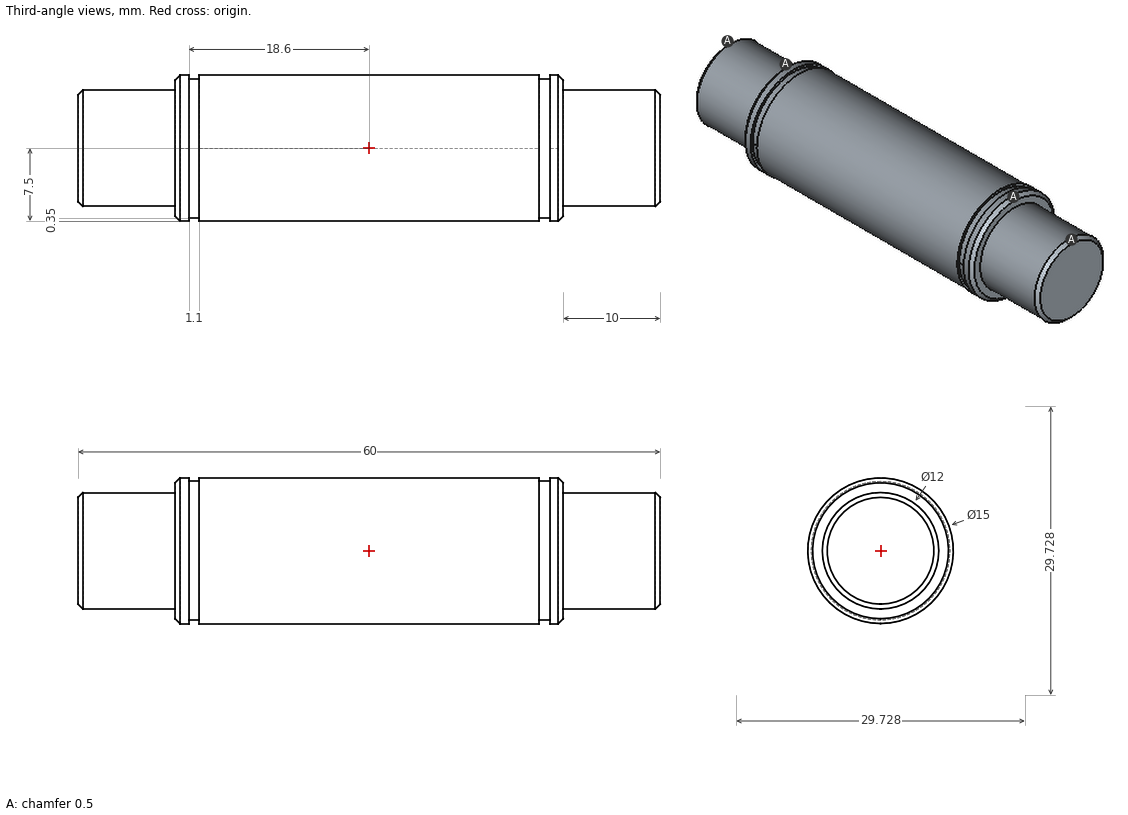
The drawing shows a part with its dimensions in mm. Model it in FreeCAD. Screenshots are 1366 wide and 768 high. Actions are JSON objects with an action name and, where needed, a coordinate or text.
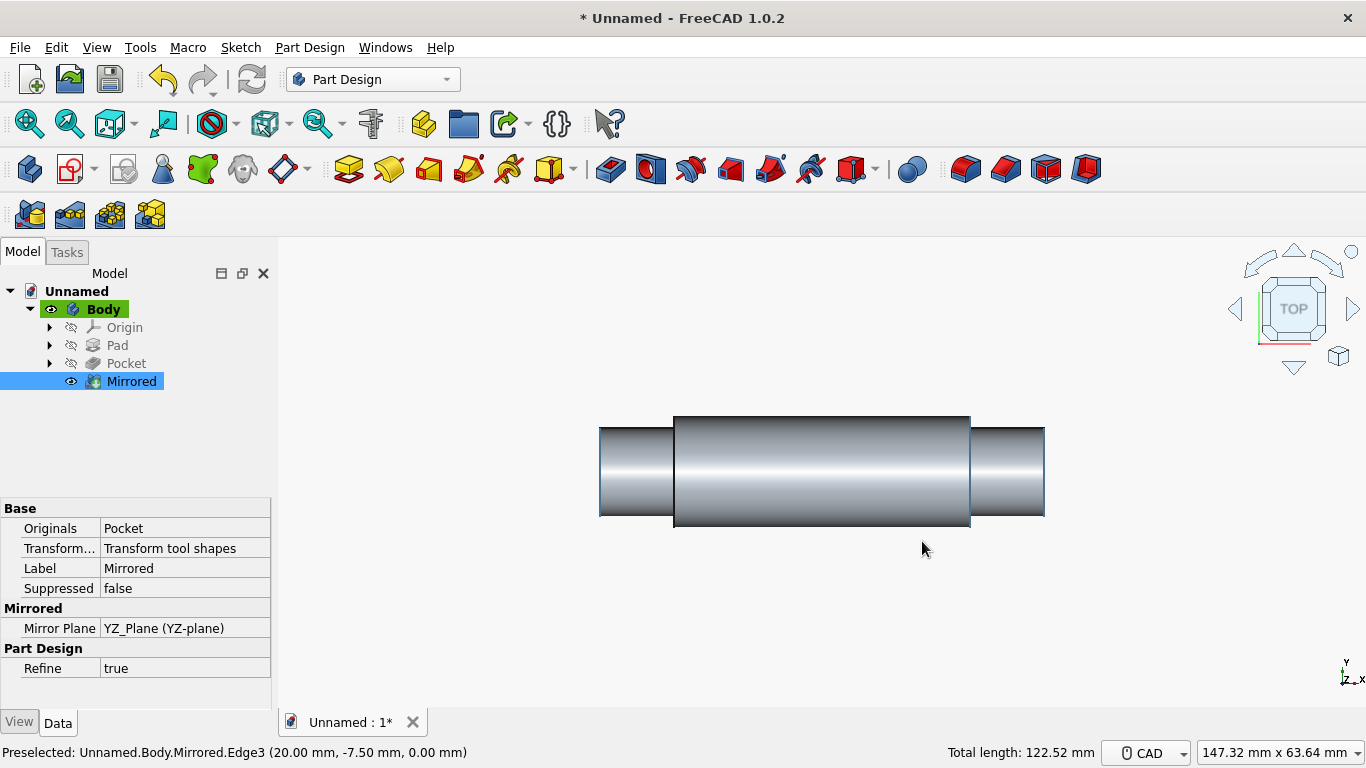
{"action": "key", "text": "v f"}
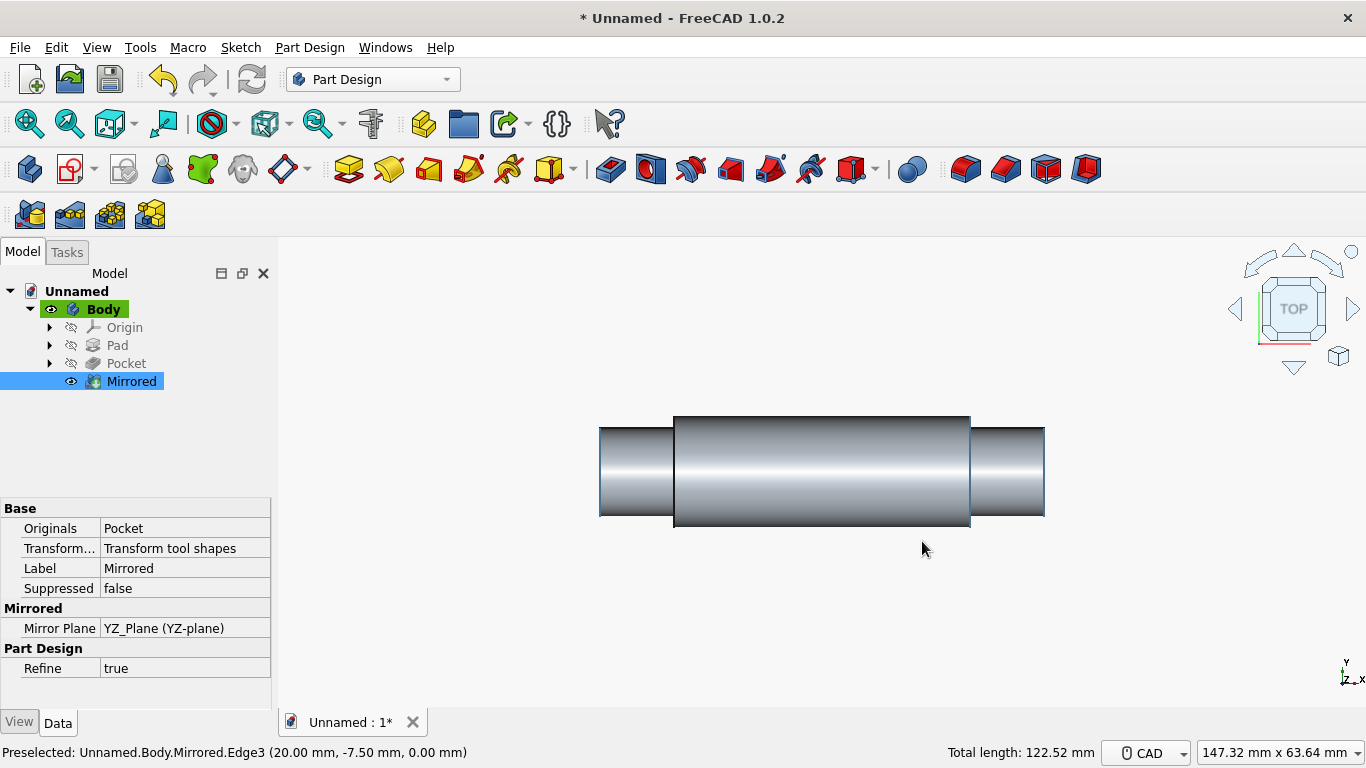
{"action": "left_click", "coordinate": [674, 516], "text": "ctrl"}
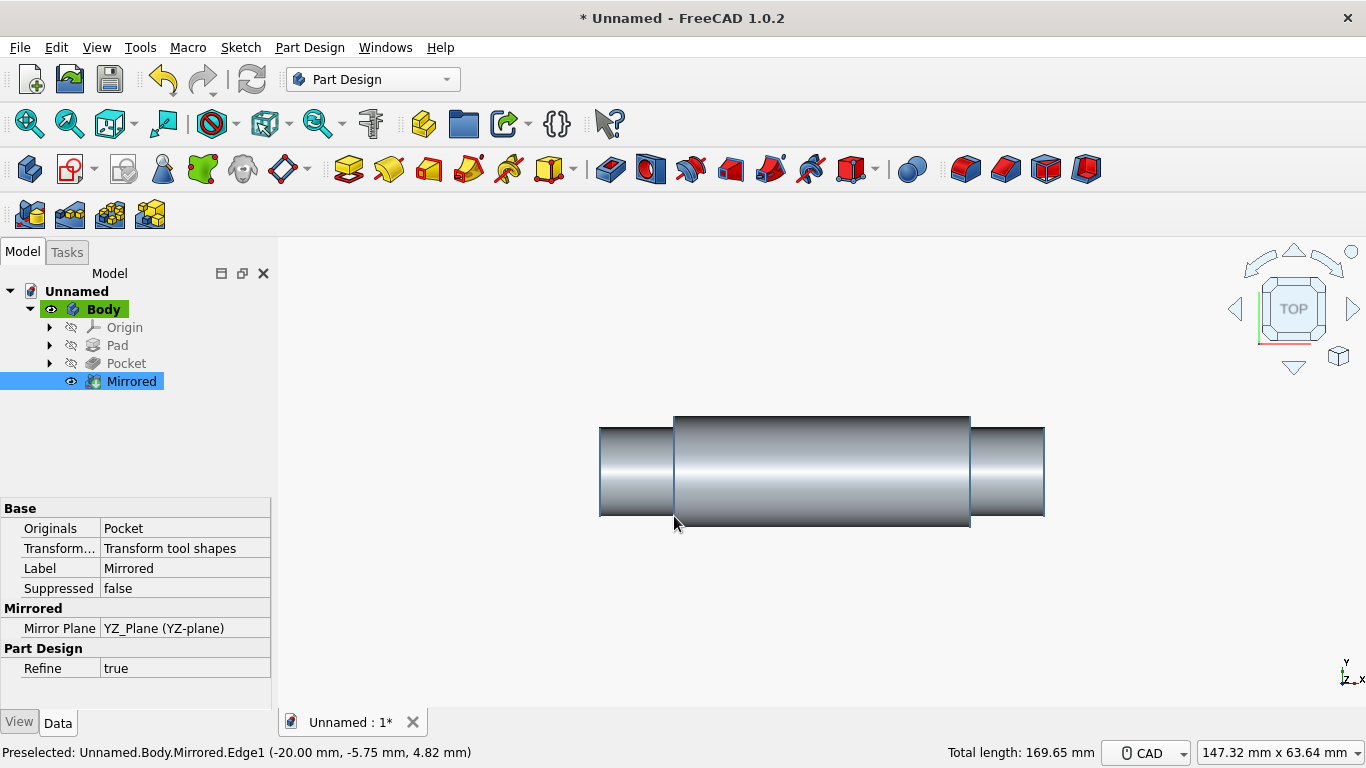
{"action": "left_click", "coordinate": [1006, 170]}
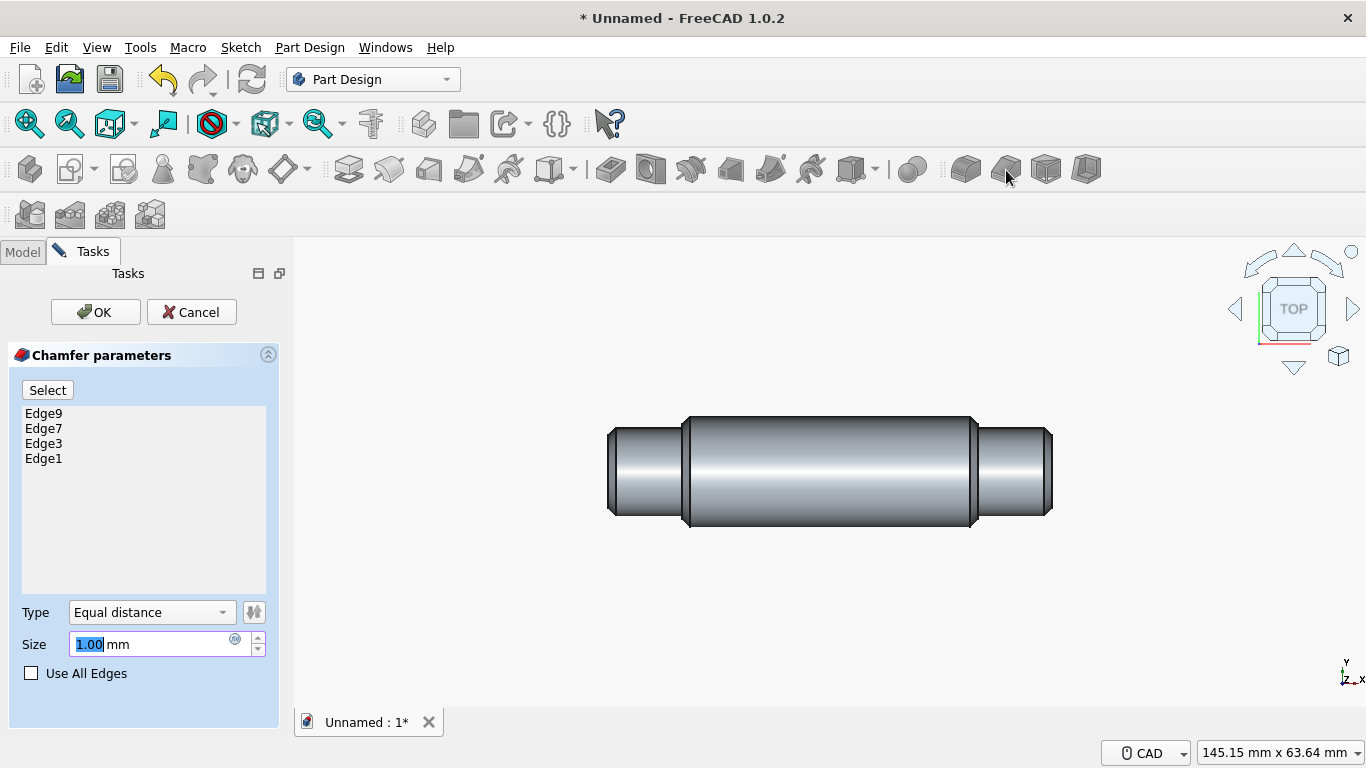
{"action": "type", "text": "0.5"}
{"action": "key", "text": "Tab"}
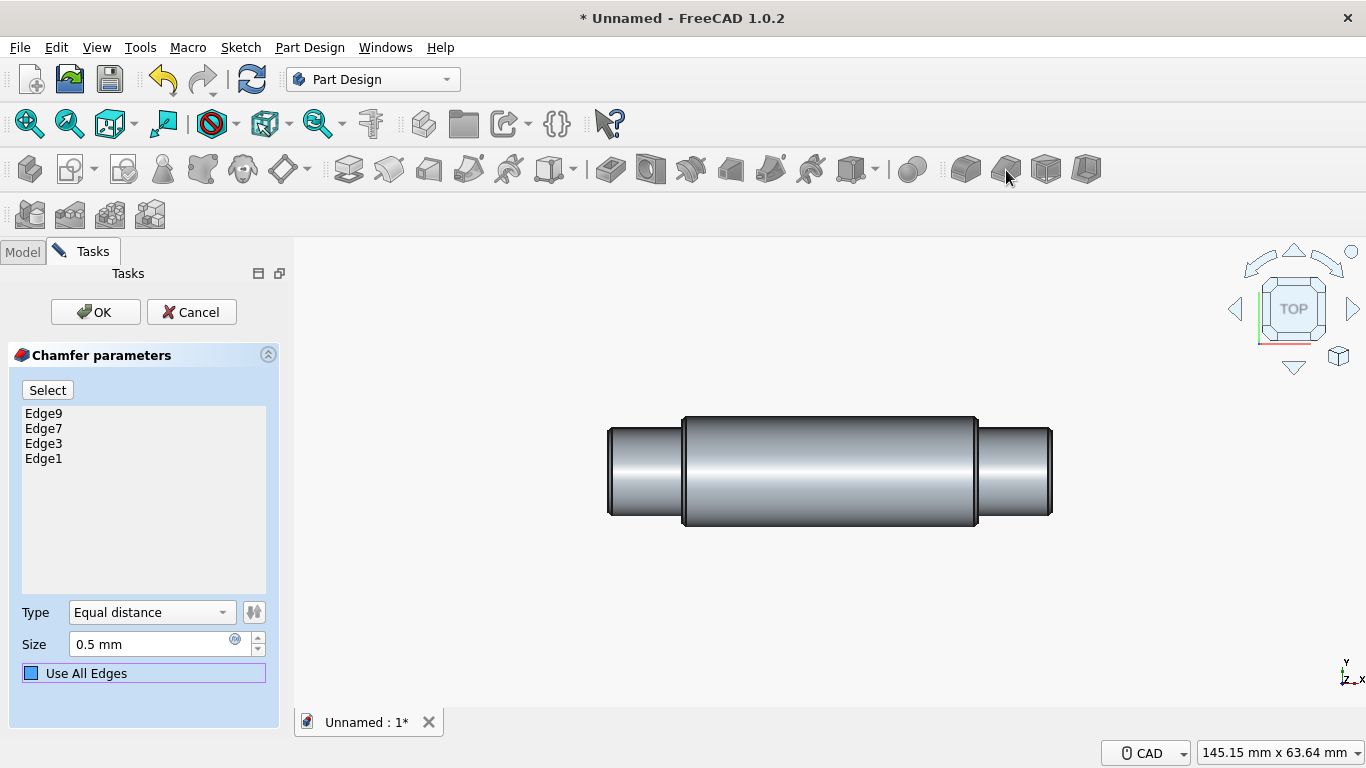
{"action": "left_click", "coordinate": [96, 312]}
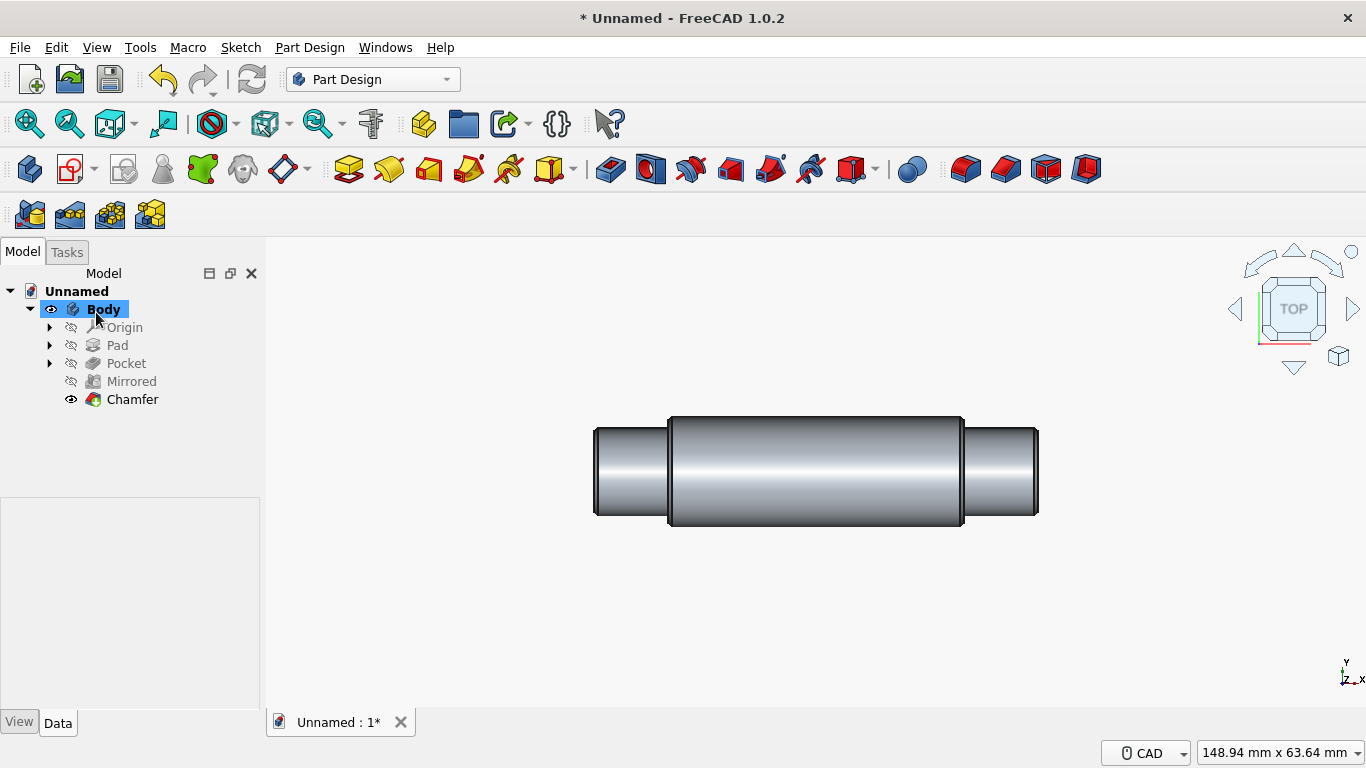
{"action": "key", "text": "v f"}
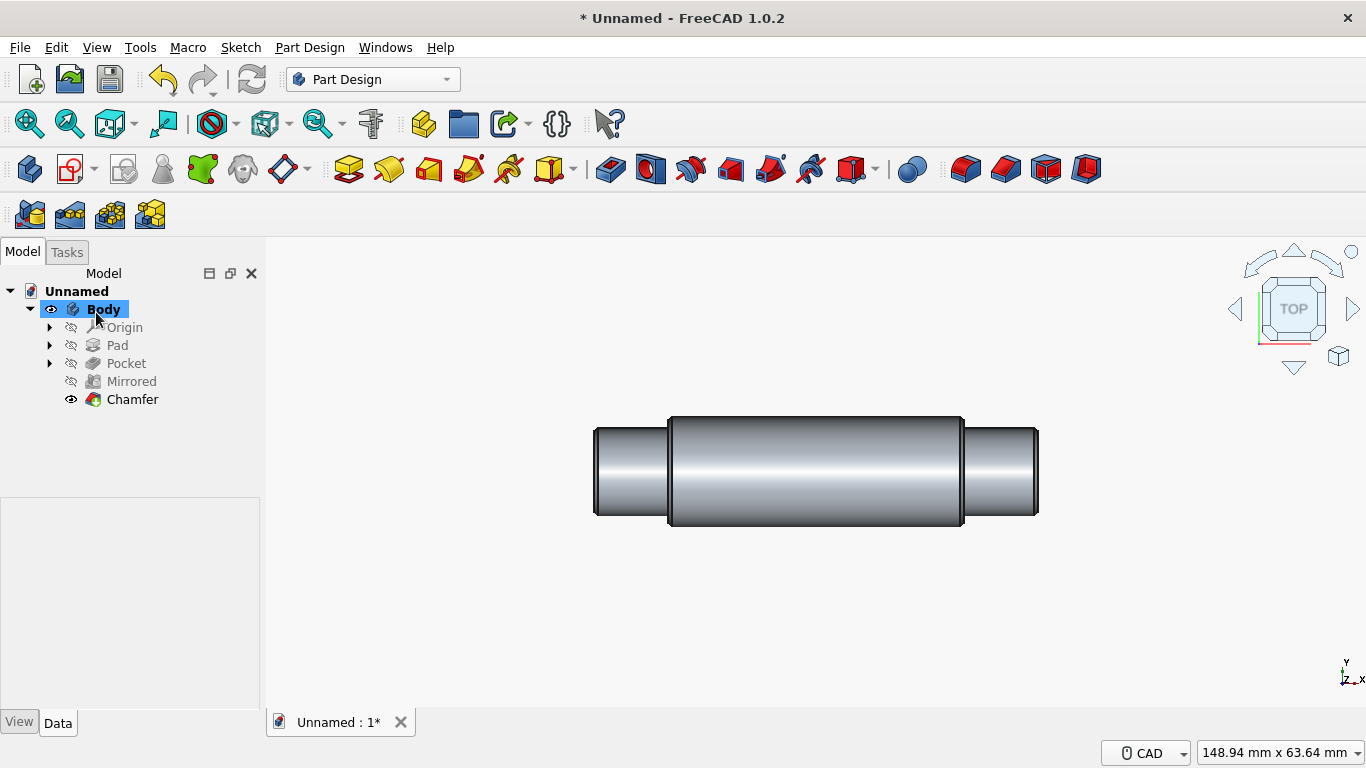
{"action": "left_click", "coordinate": [70, 170]}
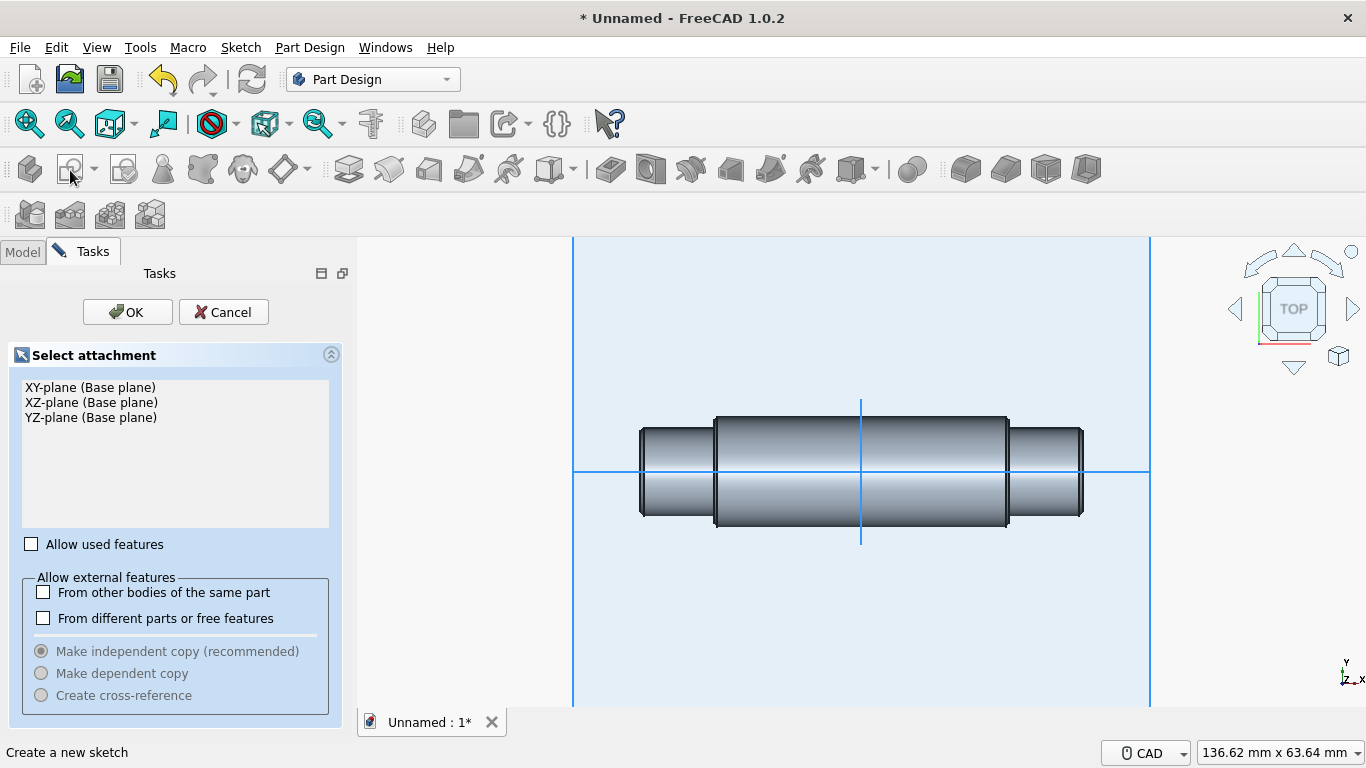
{"action": "left_click", "coordinate": [82, 388]}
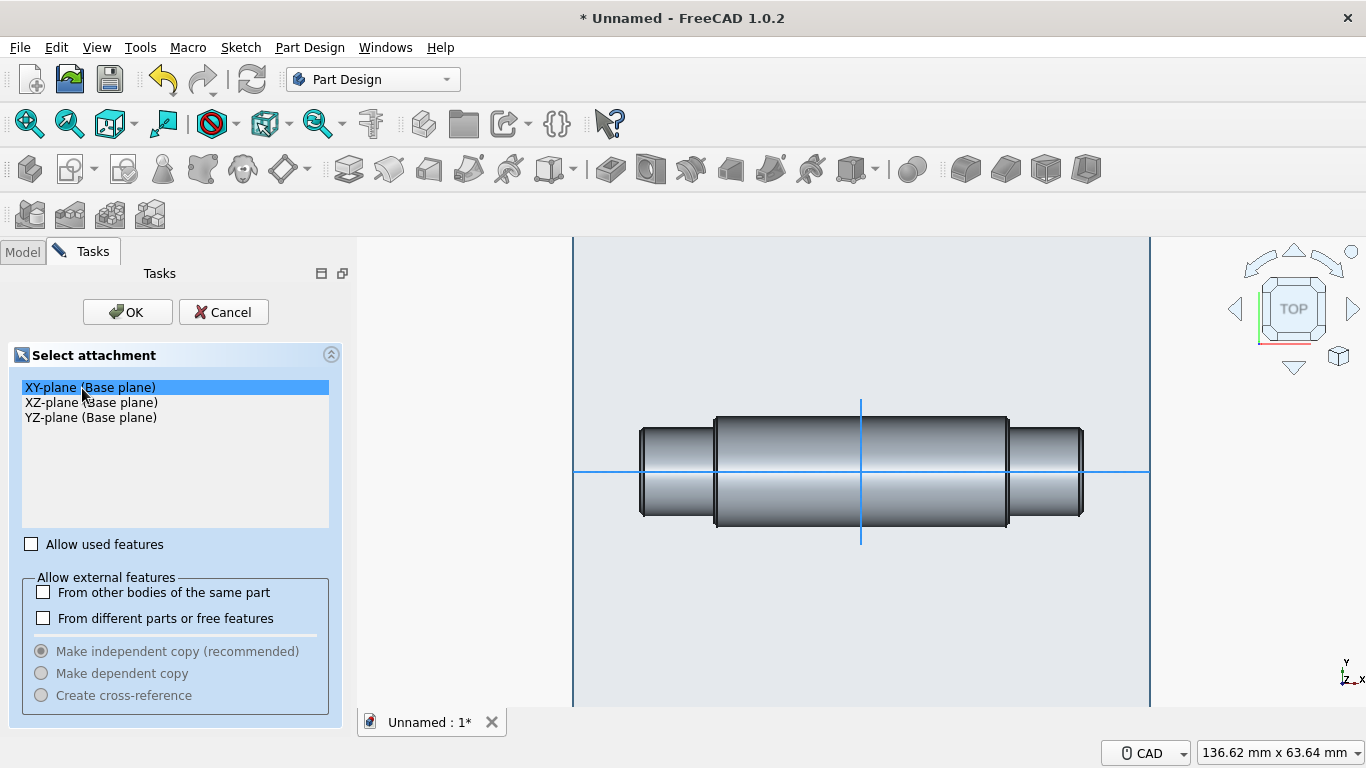
{"action": "left_click", "coordinate": [128, 312]}